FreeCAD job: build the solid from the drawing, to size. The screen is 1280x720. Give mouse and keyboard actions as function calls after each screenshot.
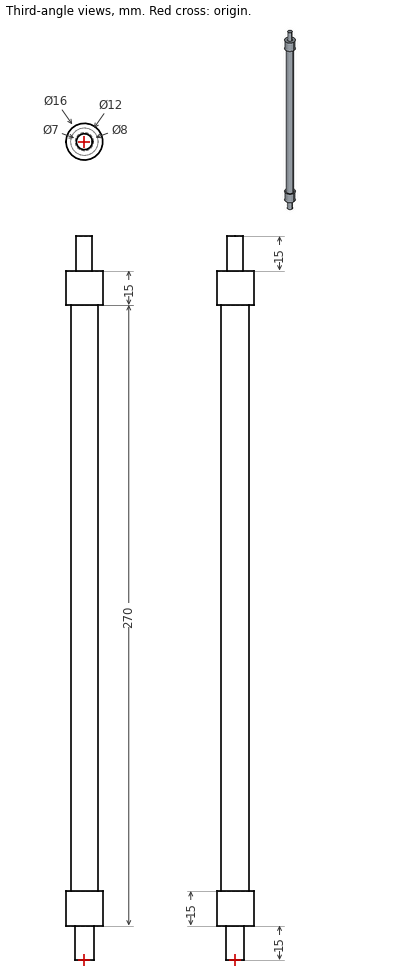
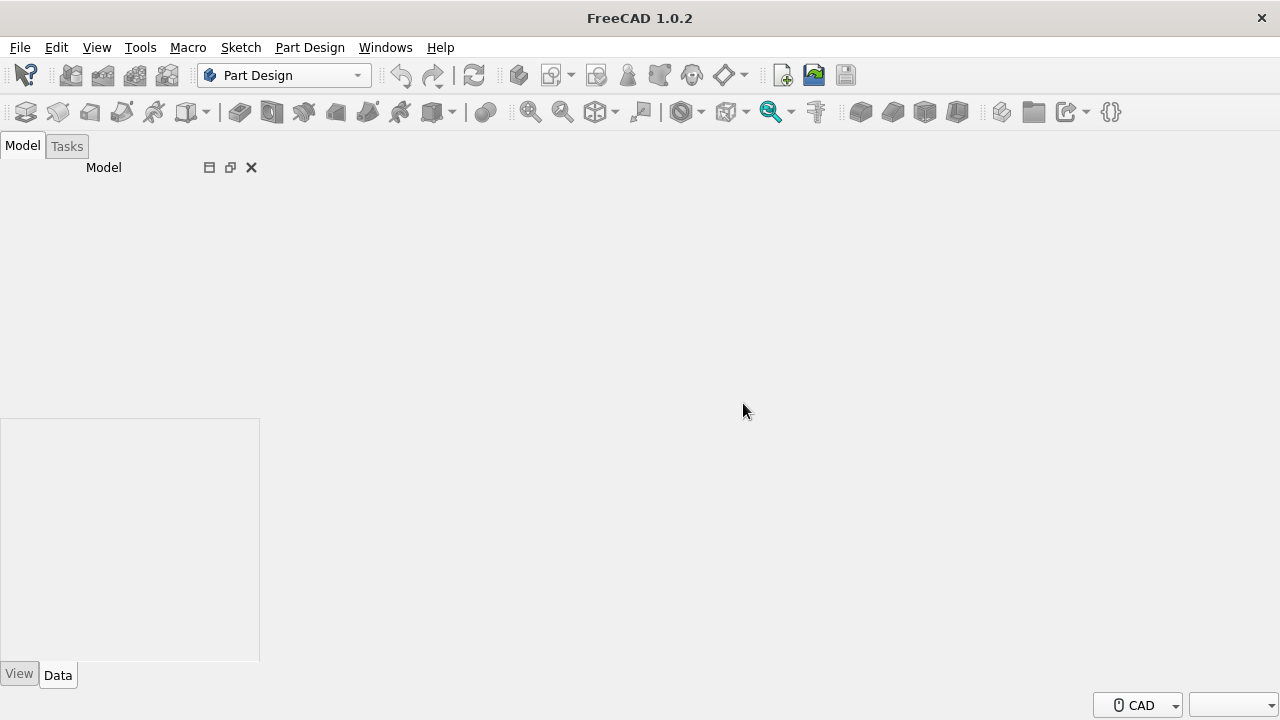
click(782, 76)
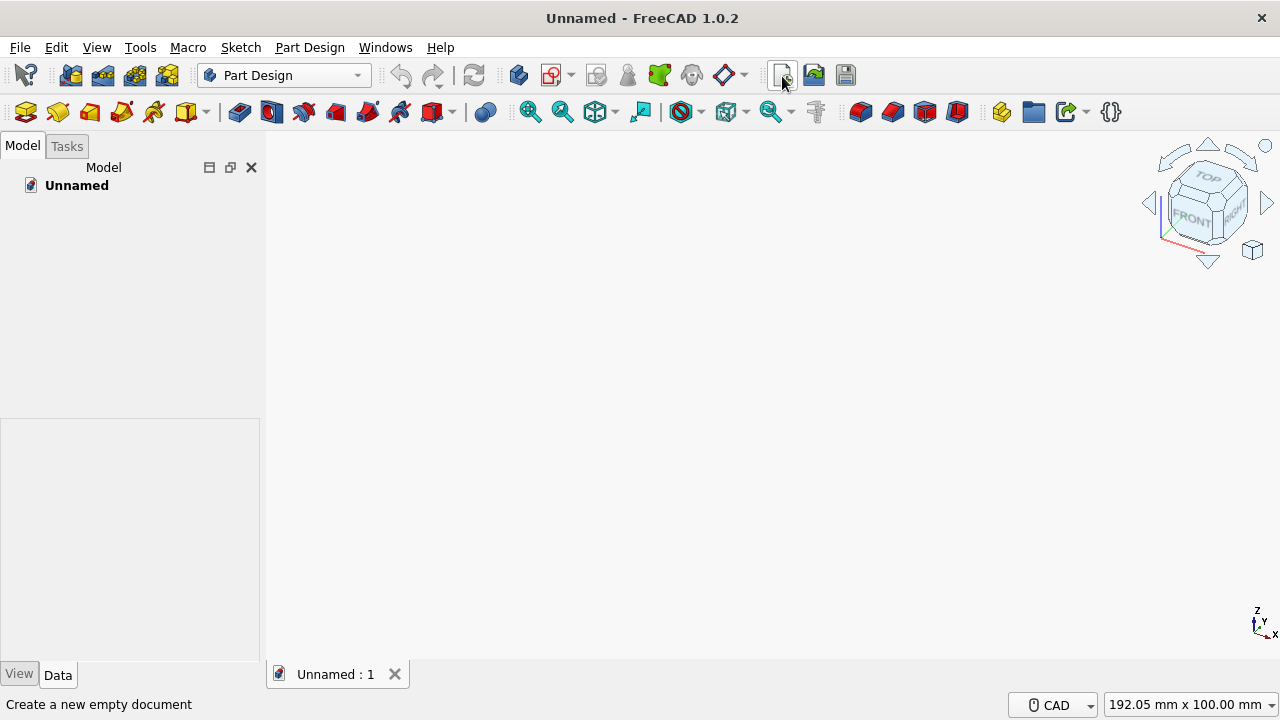
click(552, 76)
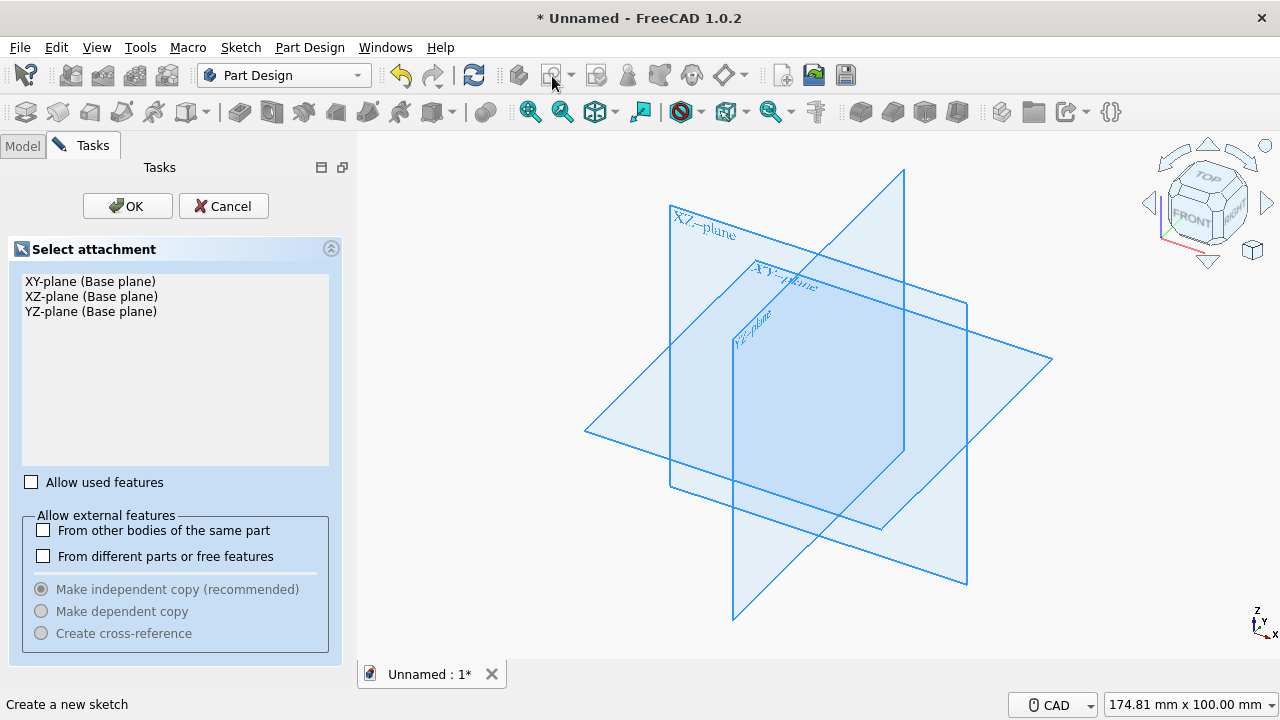
click(82, 282)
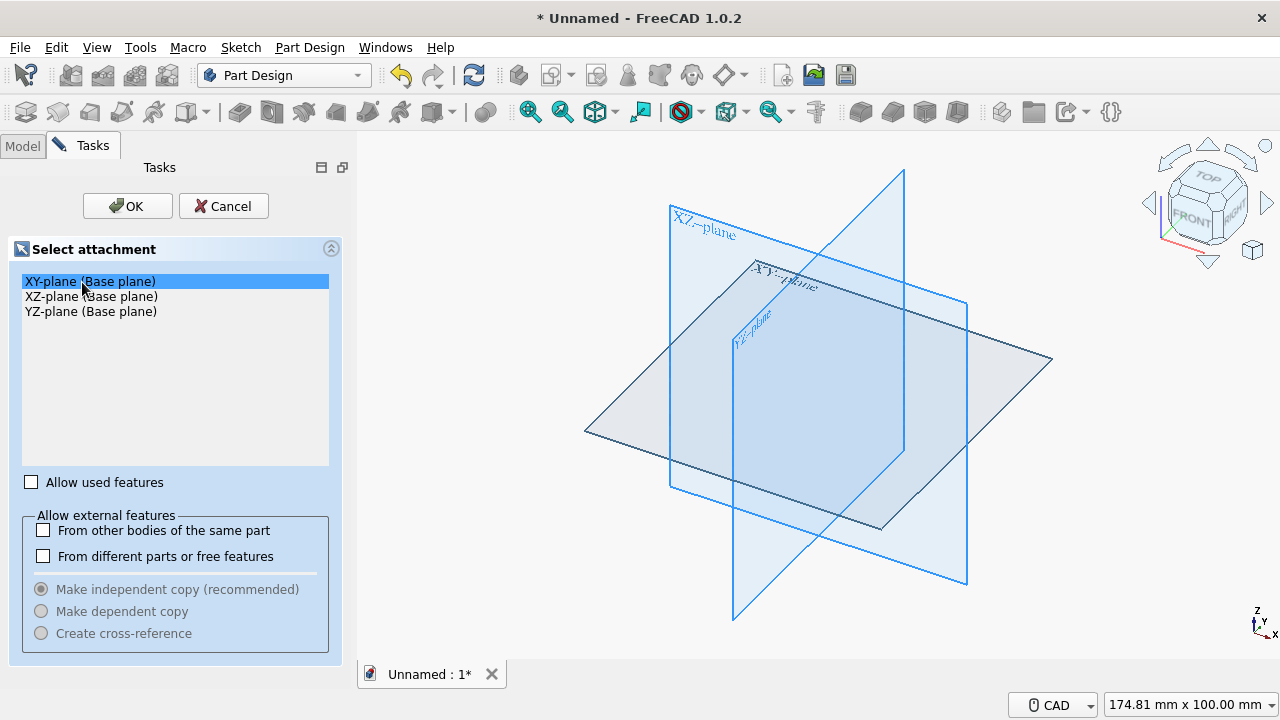
click(128, 206)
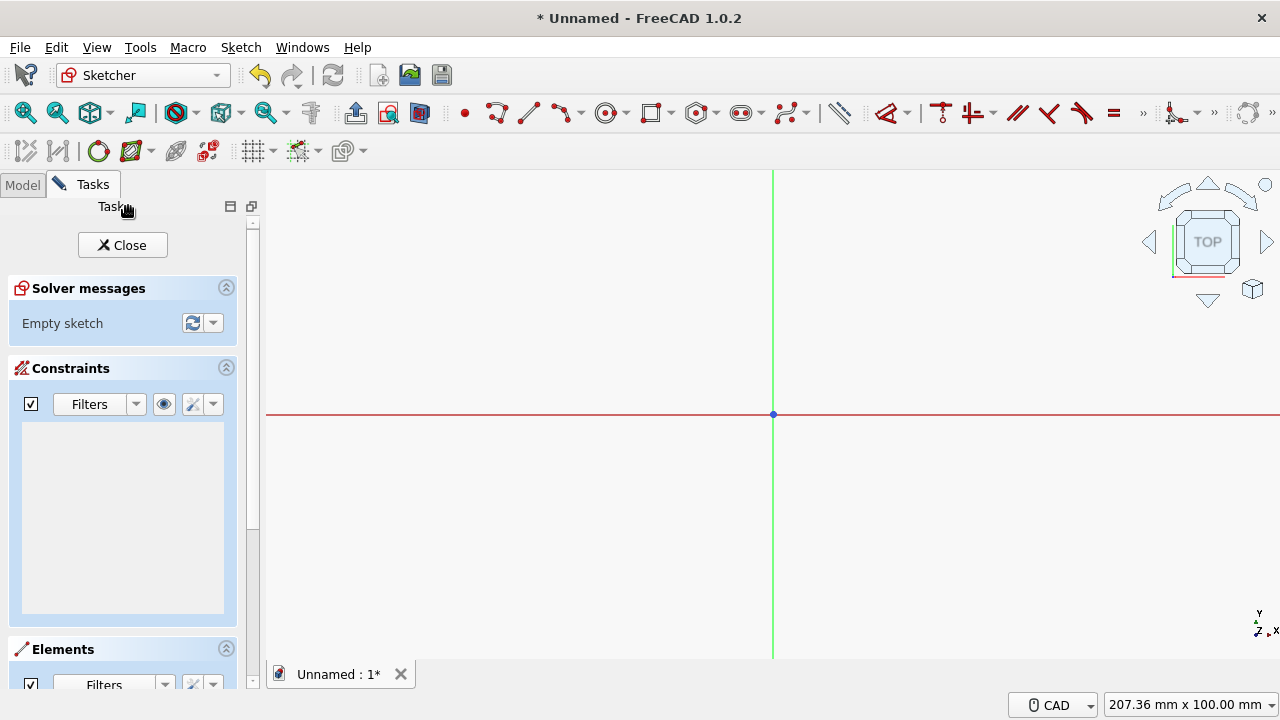
scroll(784, 414, up, 10)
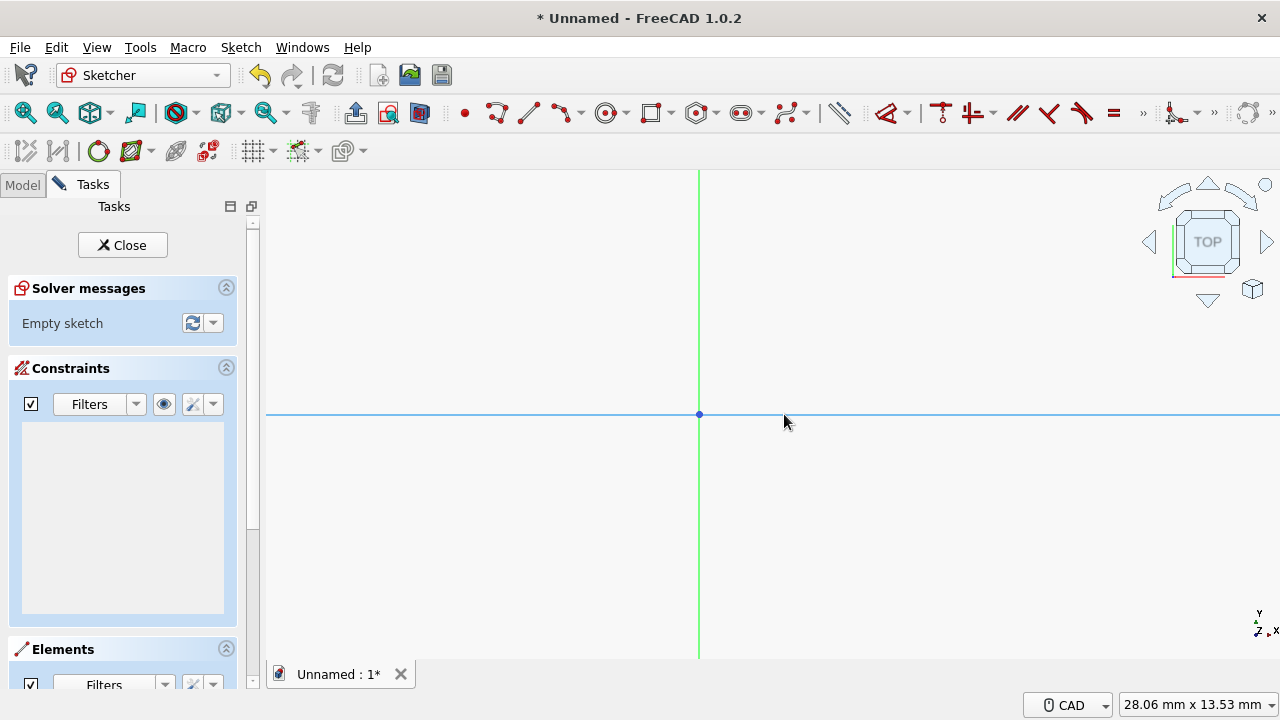
click(606, 114)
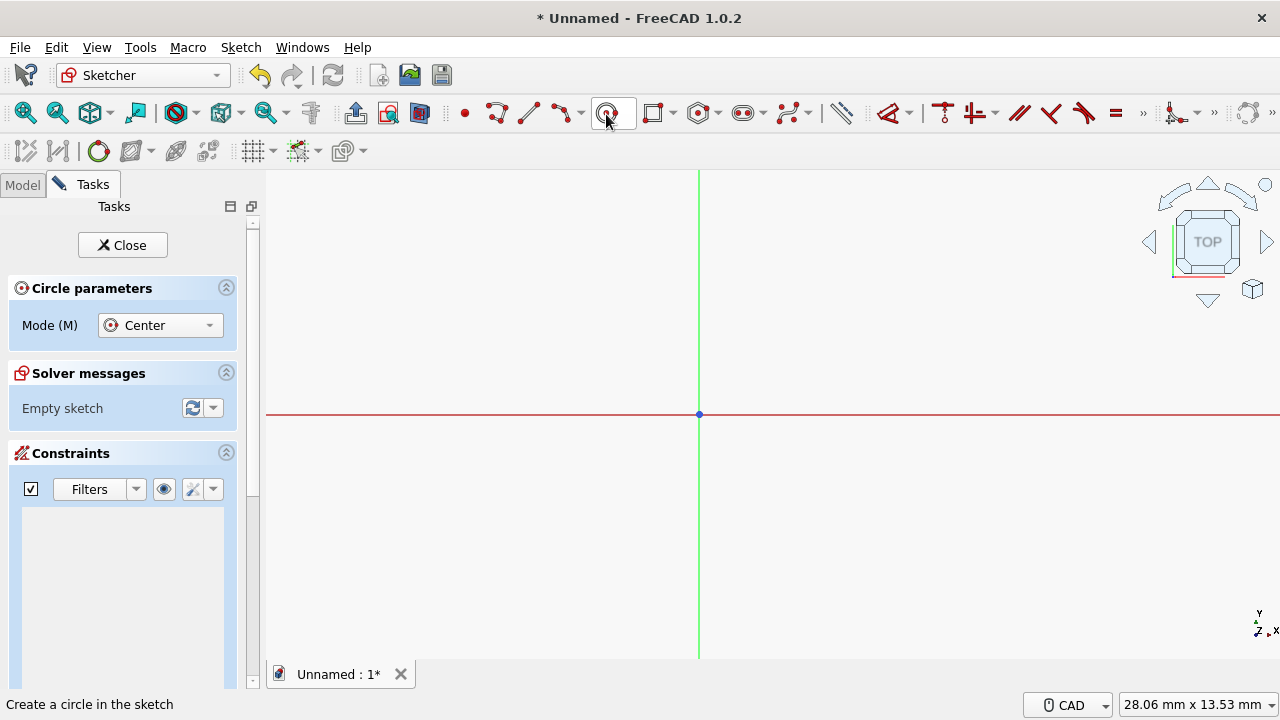
click(699, 414)
click(802, 312)
key(Escape)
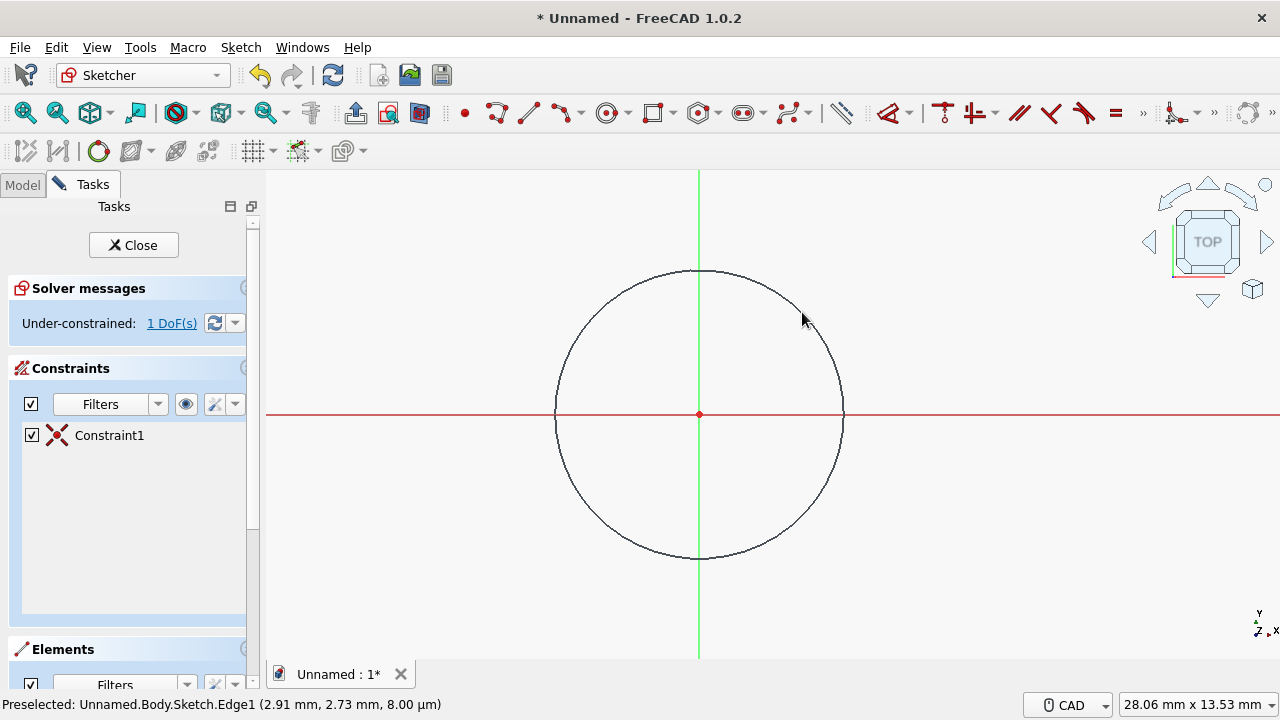
click(801, 312)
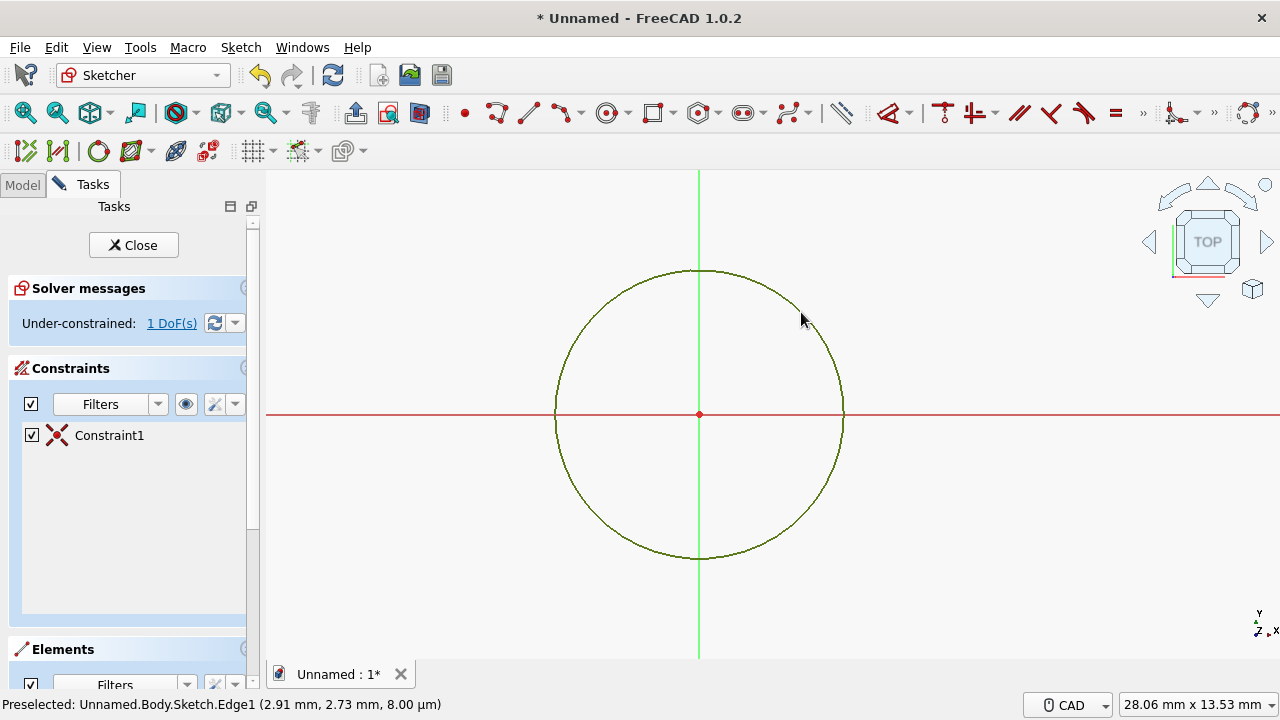
click(912, 114)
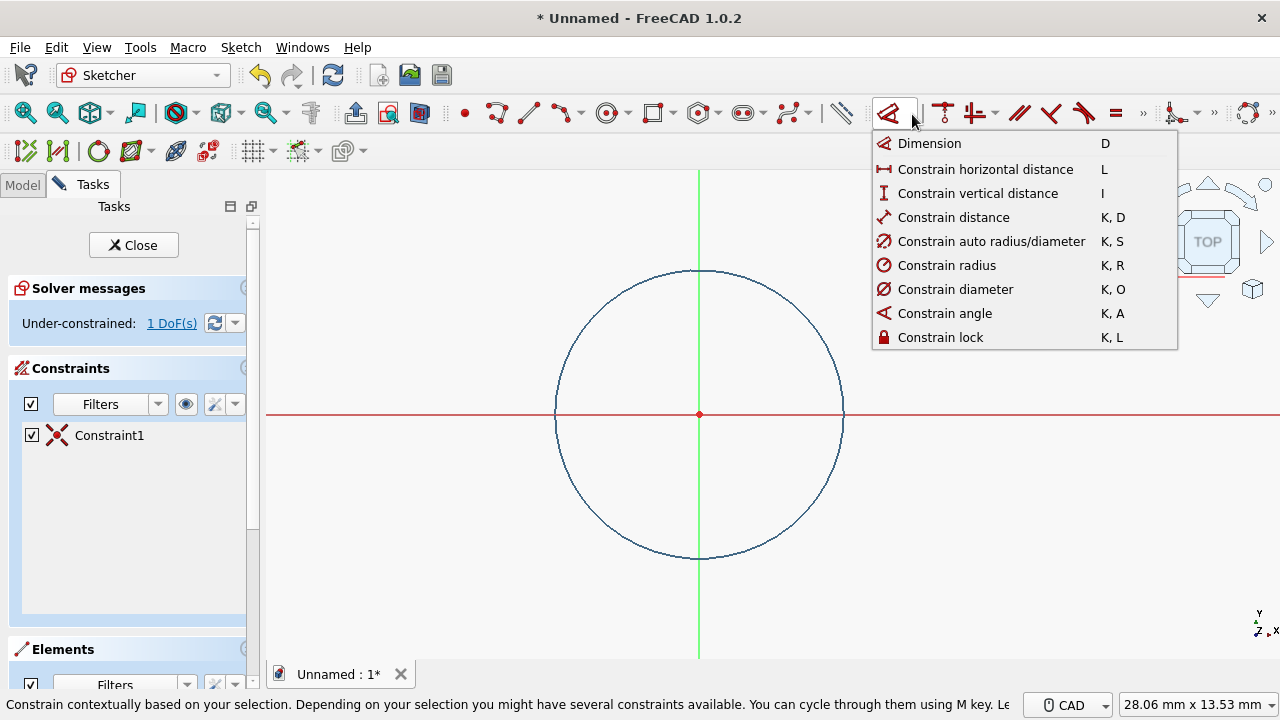
click(1025, 289)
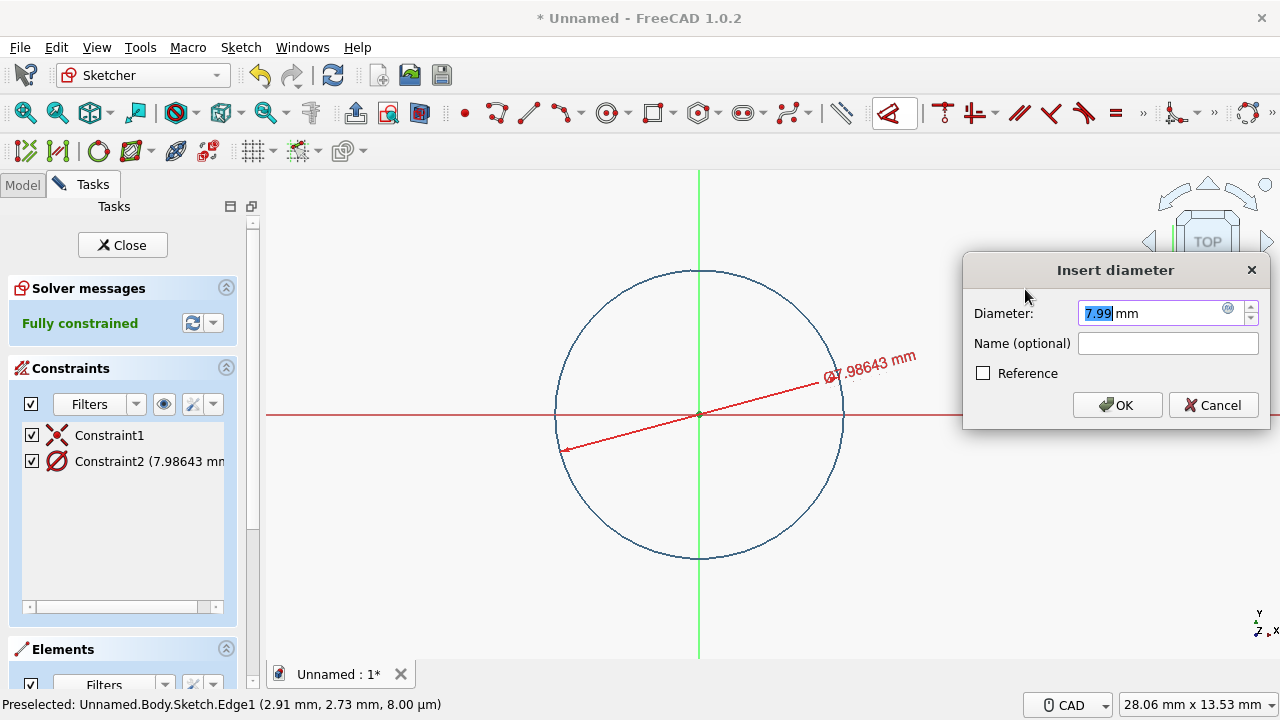
text(8)
key(Return)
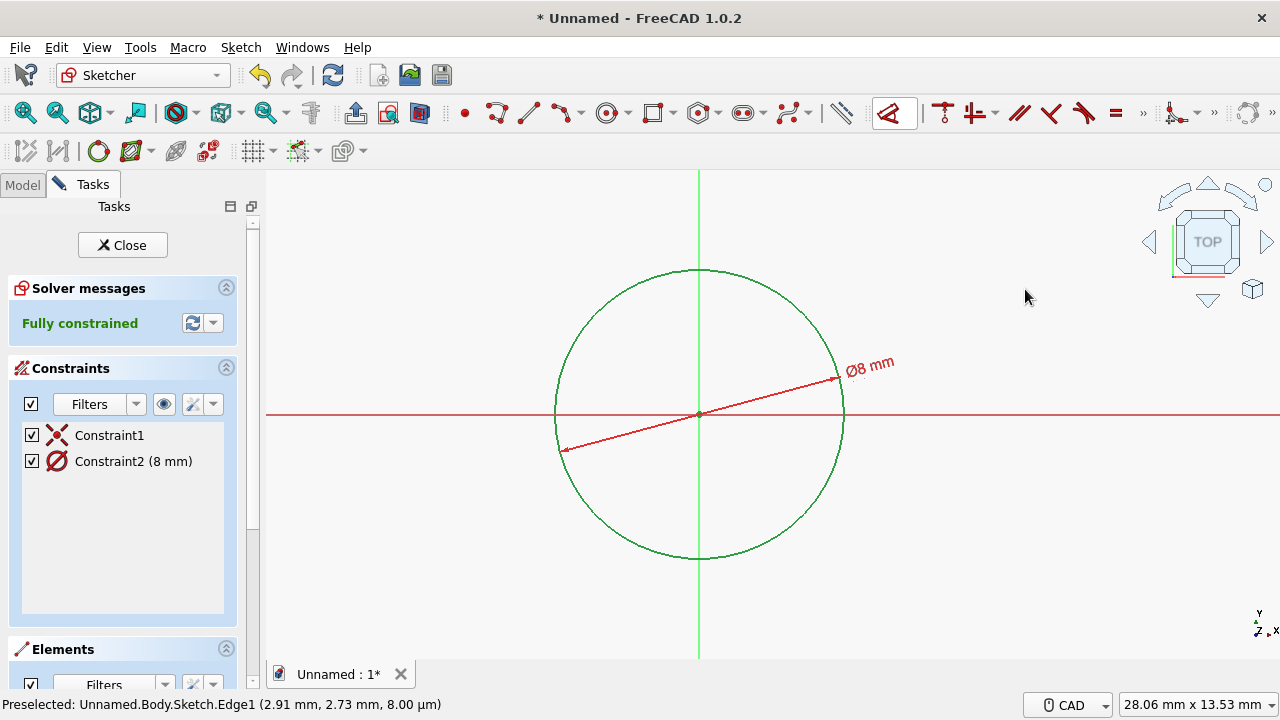
click(123, 245)